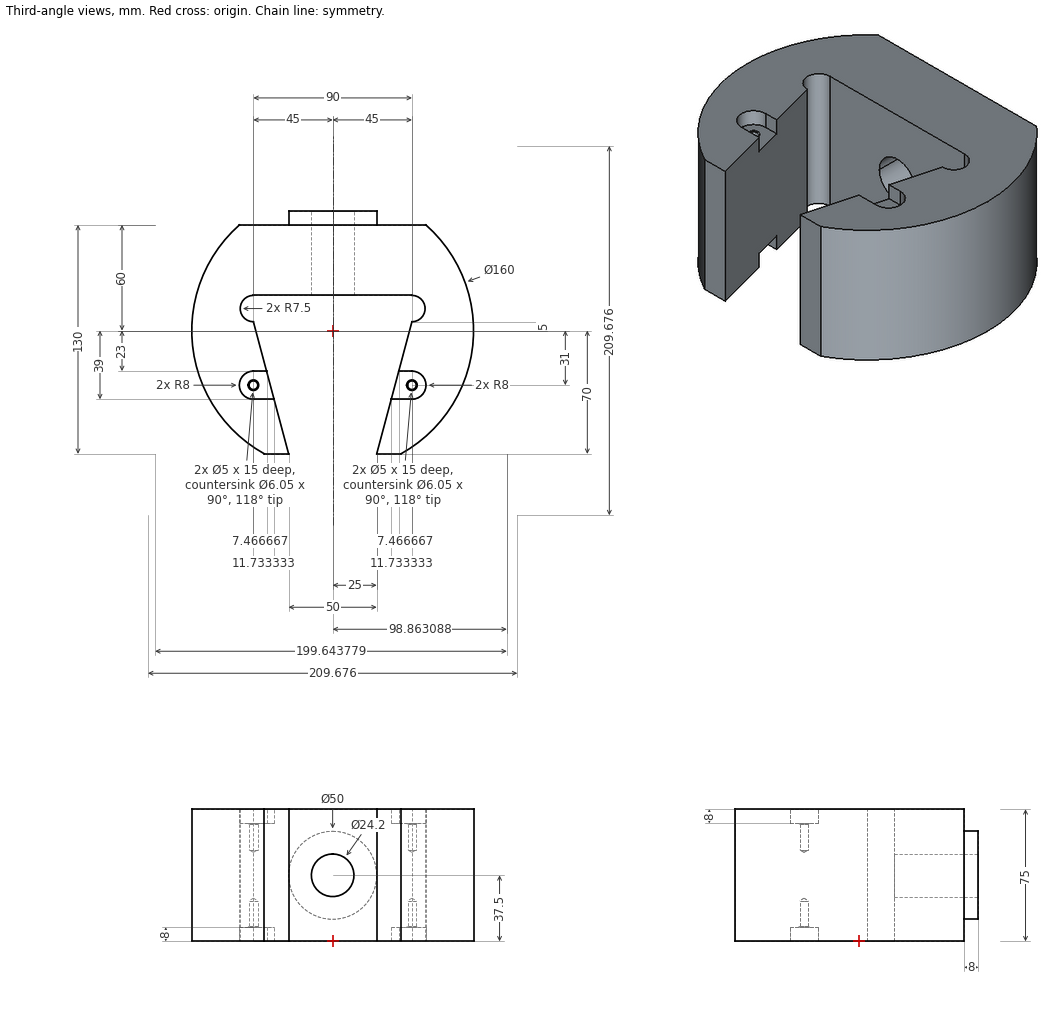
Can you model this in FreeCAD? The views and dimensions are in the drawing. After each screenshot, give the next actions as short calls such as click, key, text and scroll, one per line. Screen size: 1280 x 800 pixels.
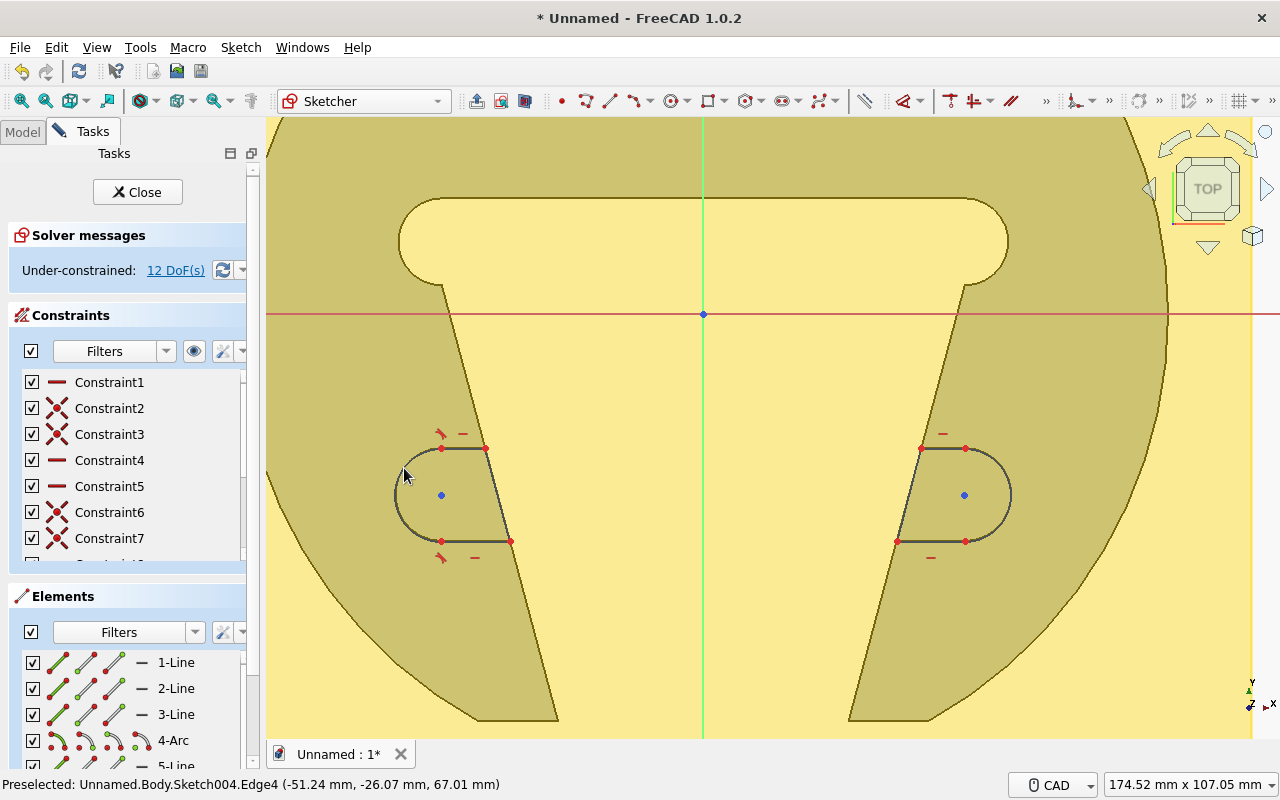
click(945, 542)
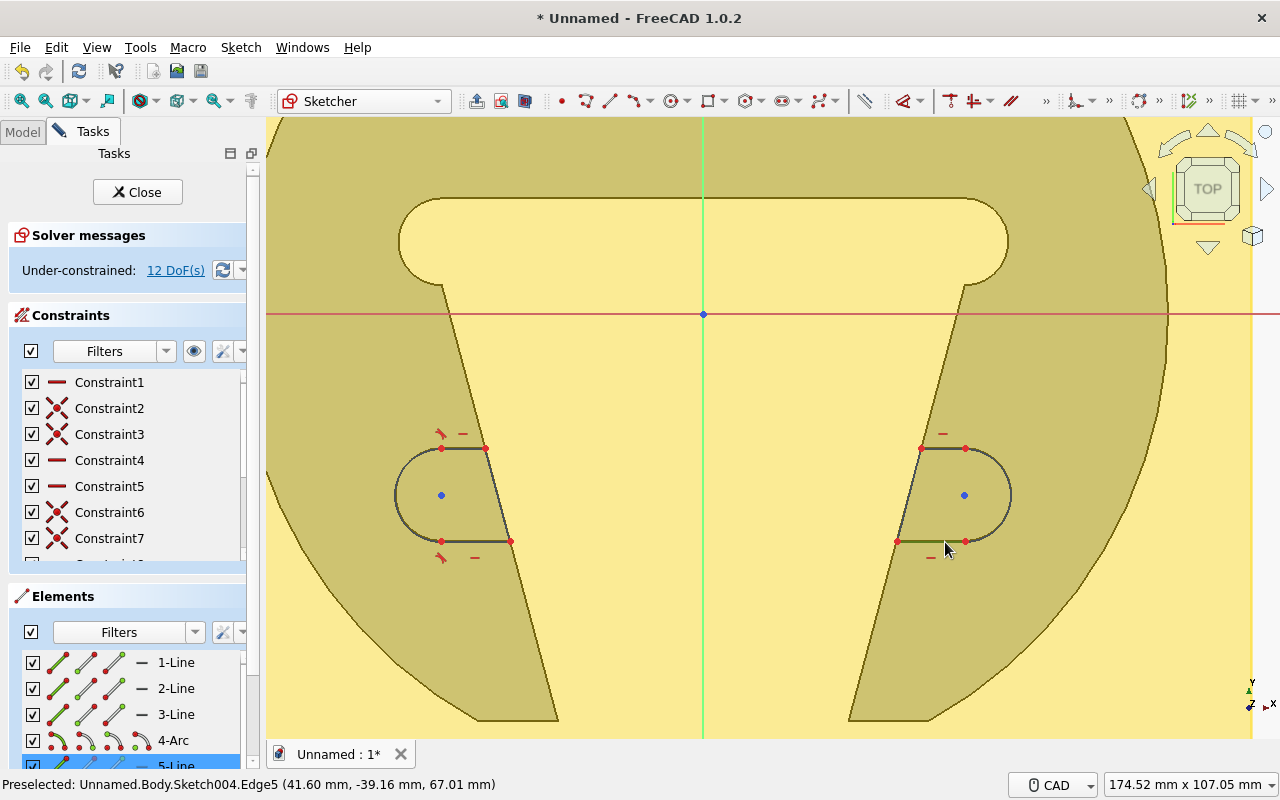
click(1002, 523)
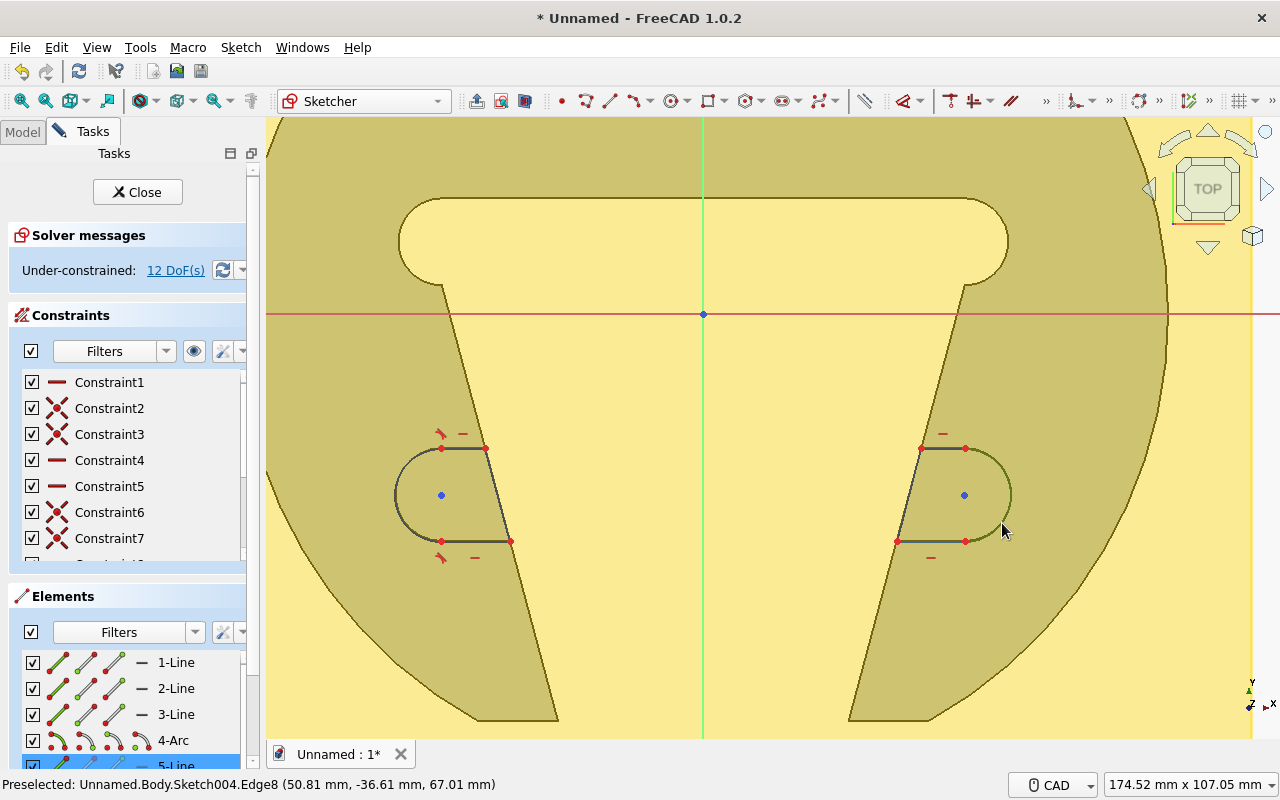
key(t)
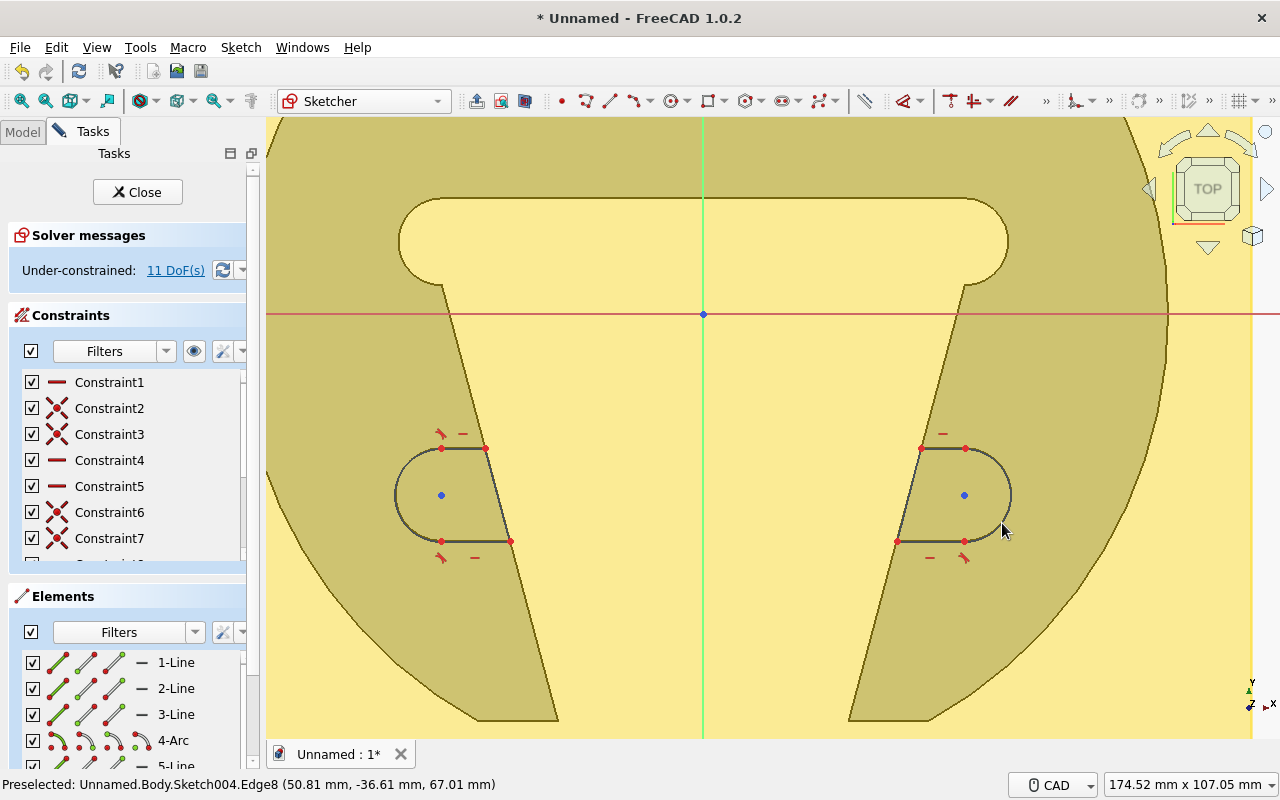
click(934, 449)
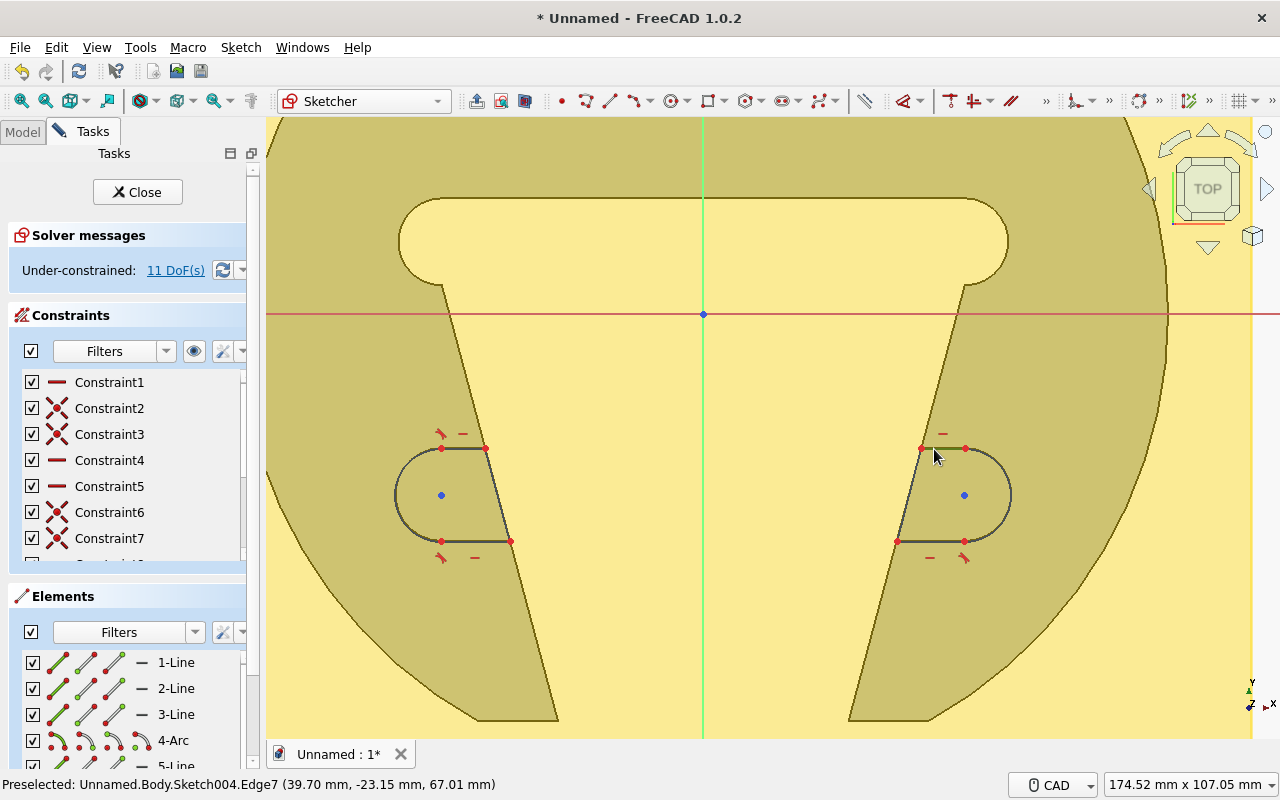
click(1002, 523)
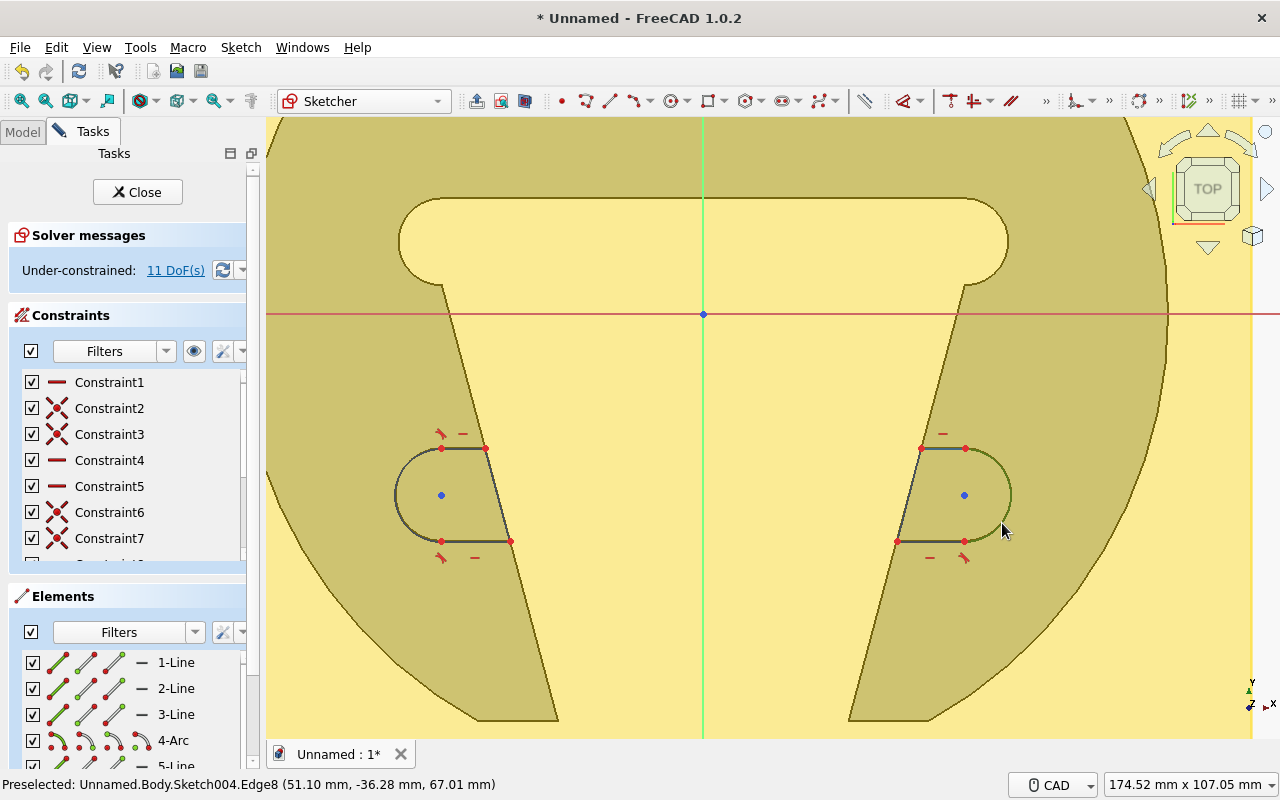
key(t)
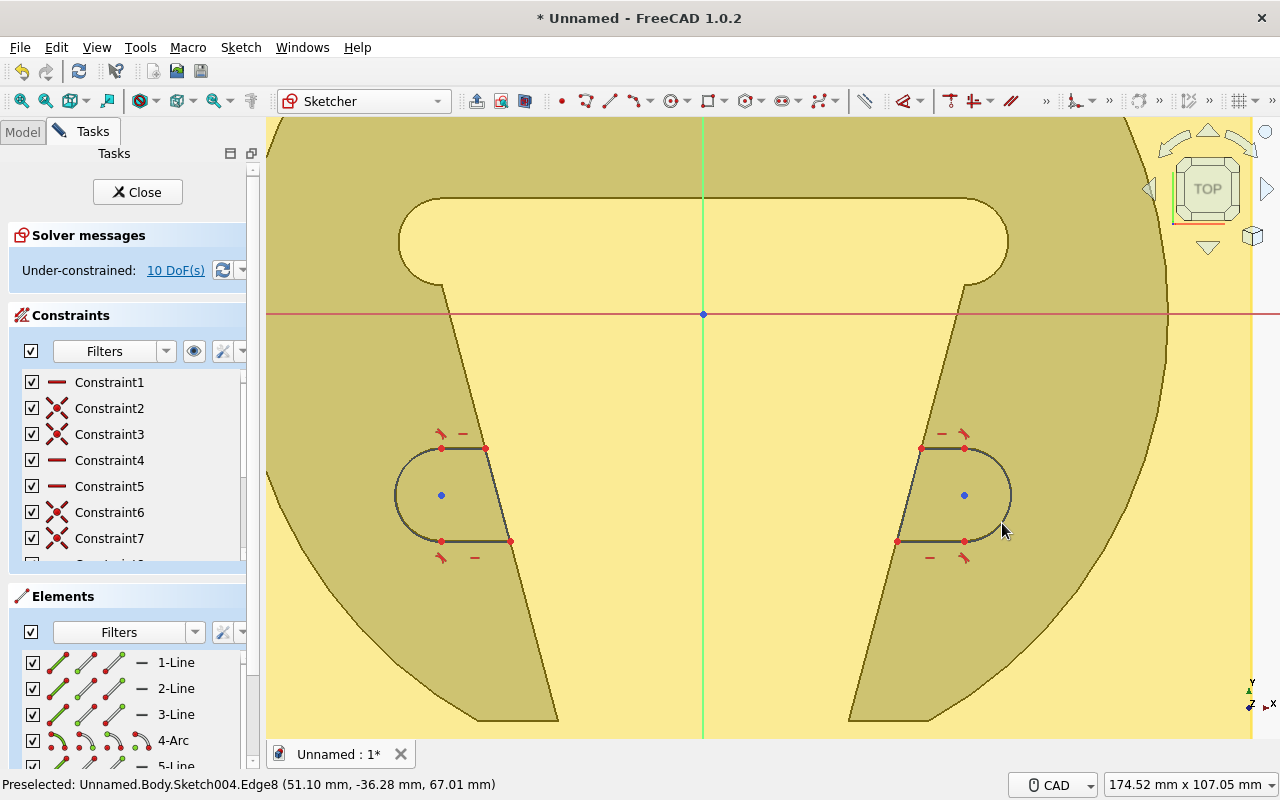
click(404, 468)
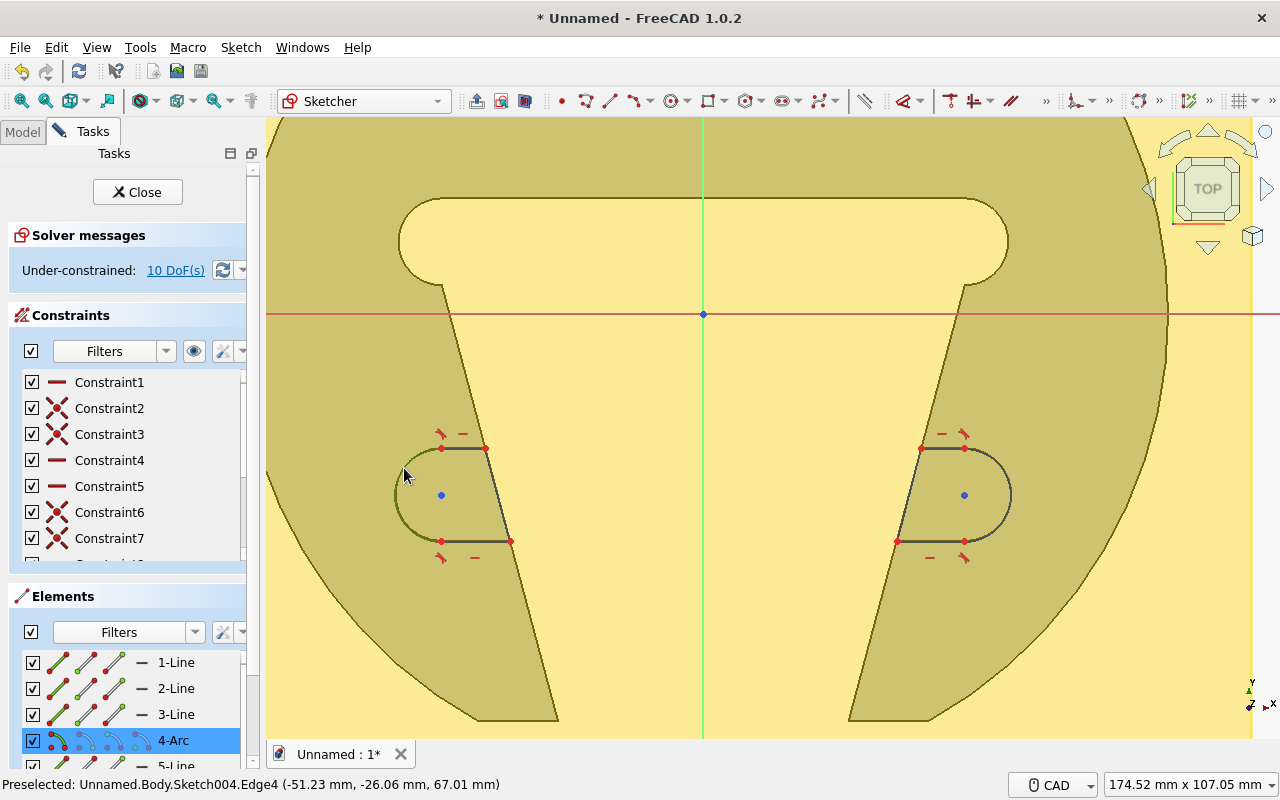
click(1002, 523)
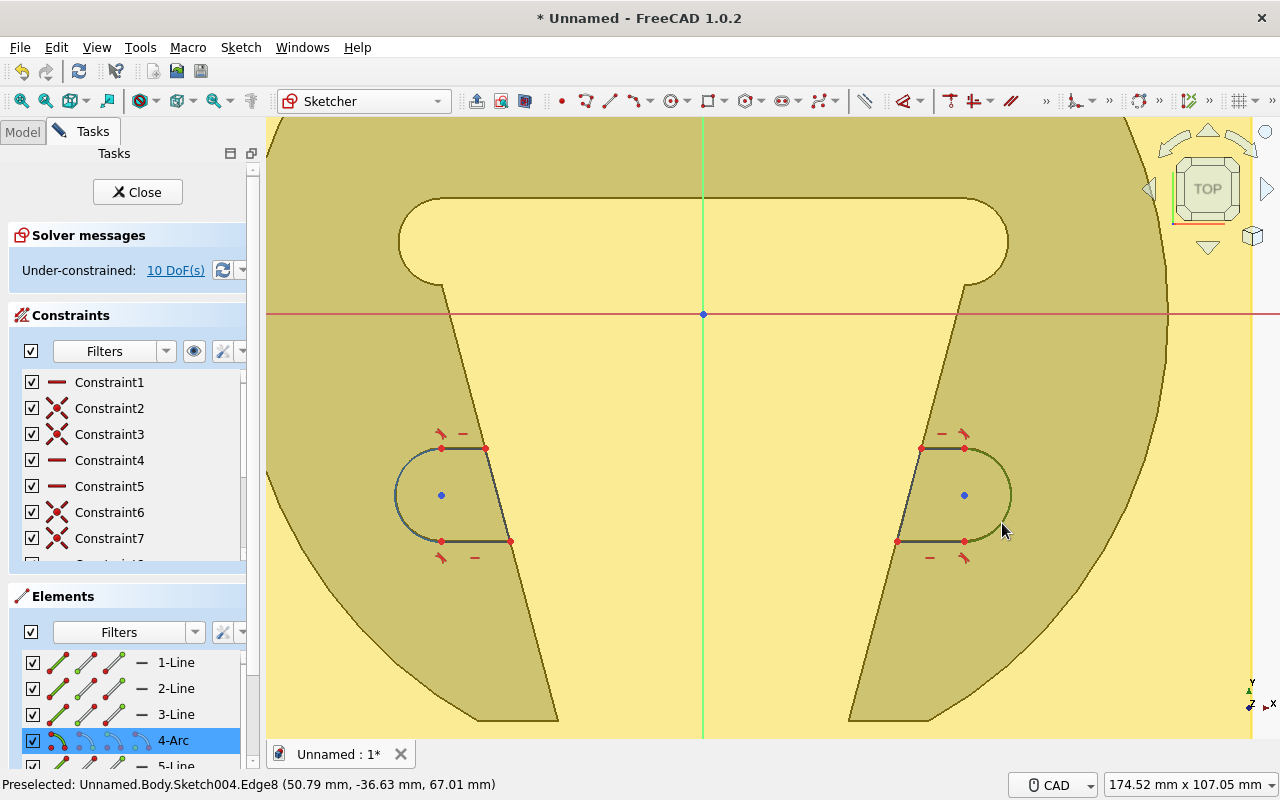
key(e)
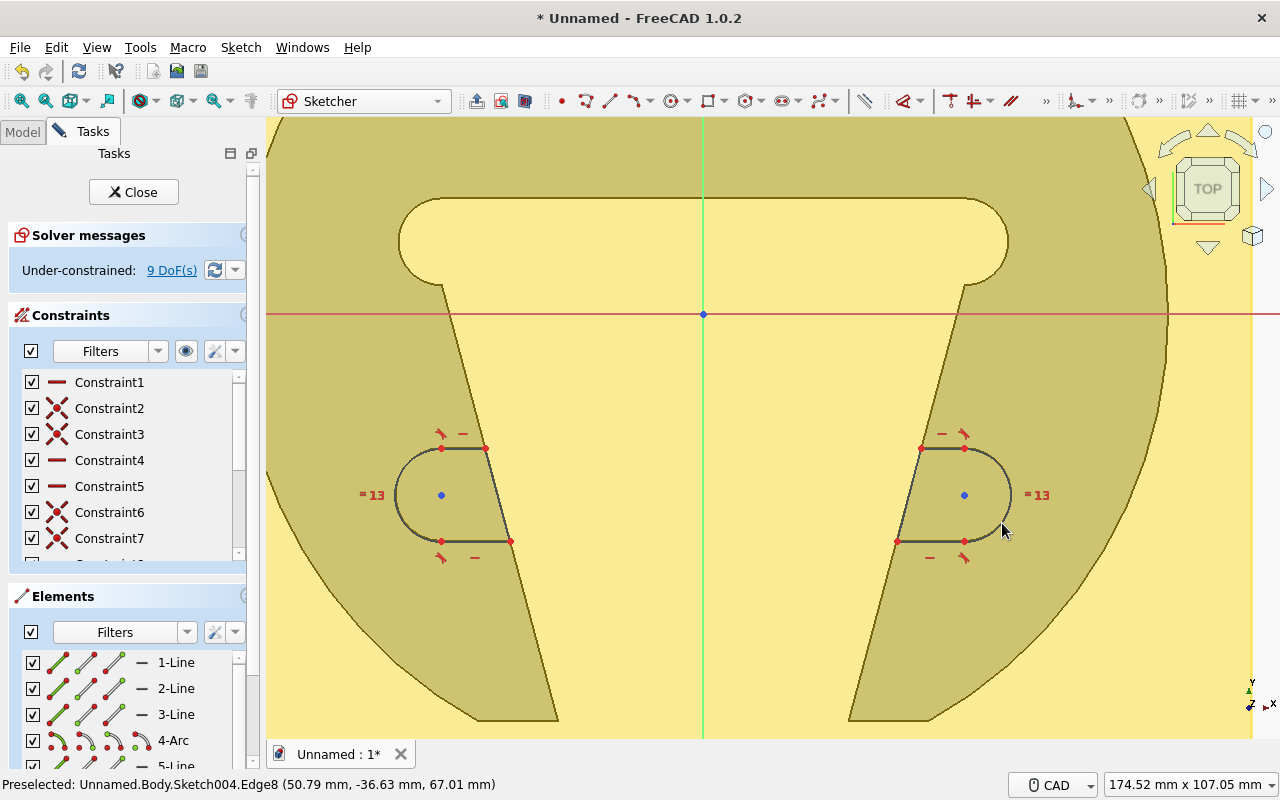
click(441, 495)